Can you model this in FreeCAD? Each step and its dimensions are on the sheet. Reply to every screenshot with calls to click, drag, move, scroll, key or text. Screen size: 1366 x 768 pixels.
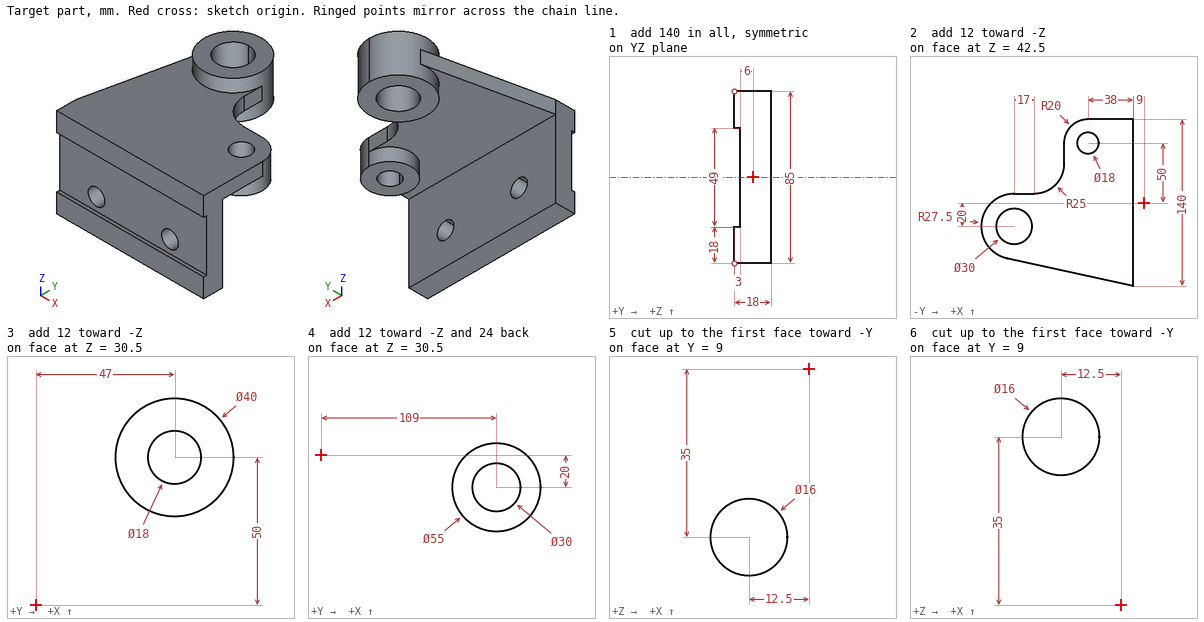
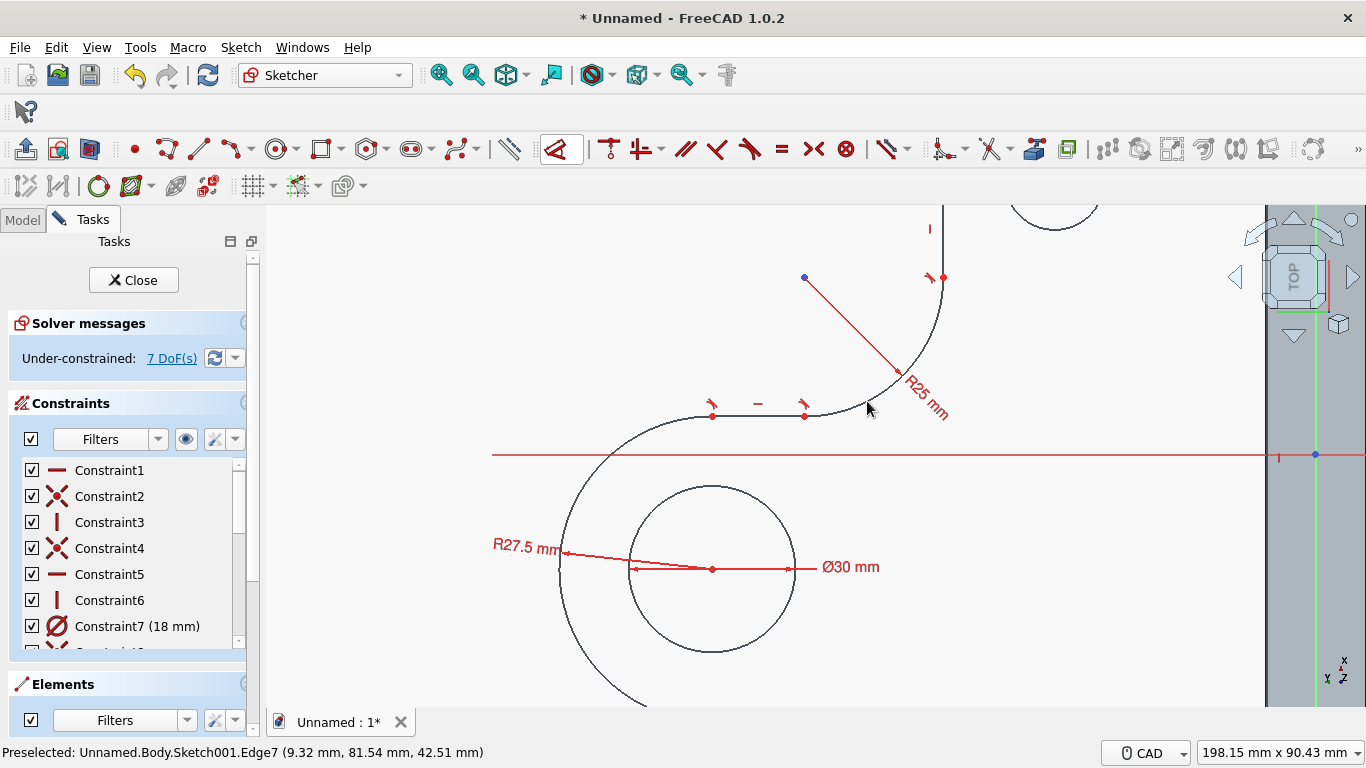
scroll(637, 457, down, 5)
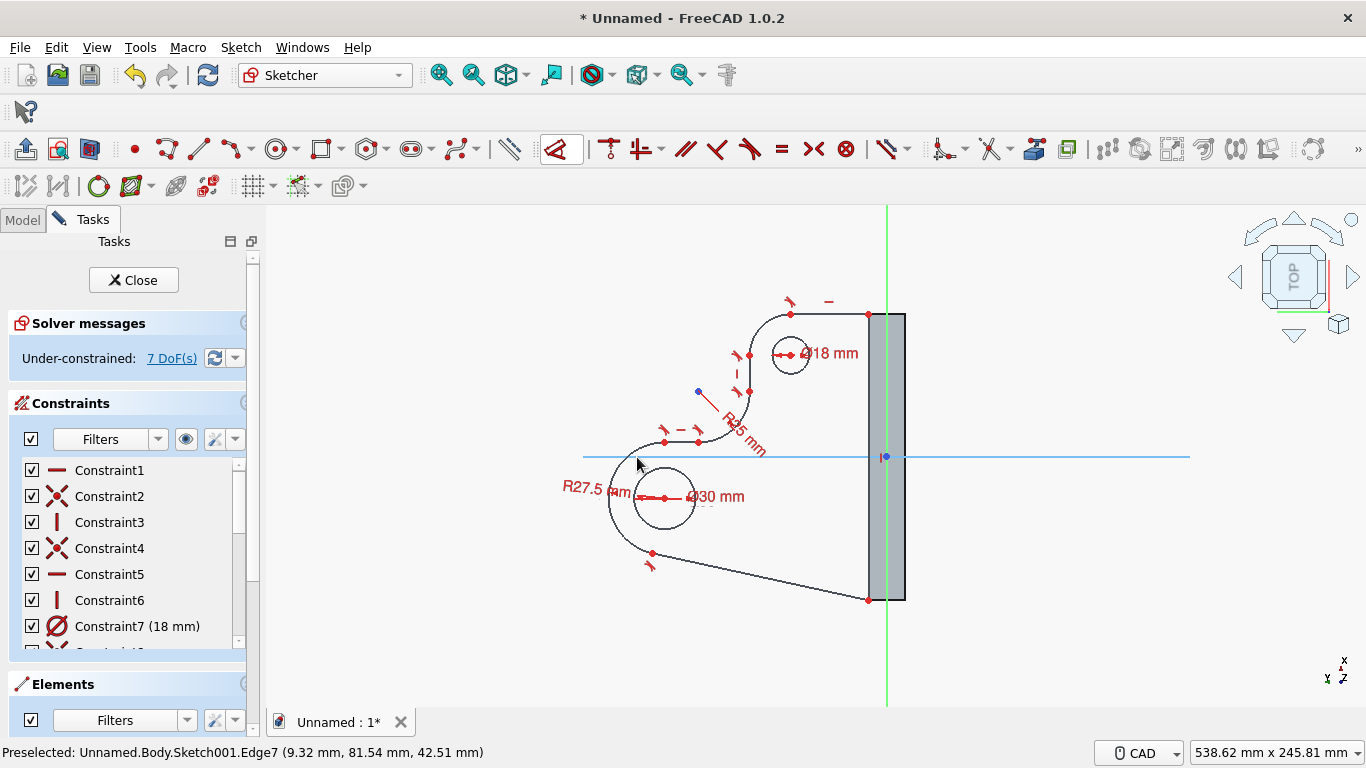
click(772, 319)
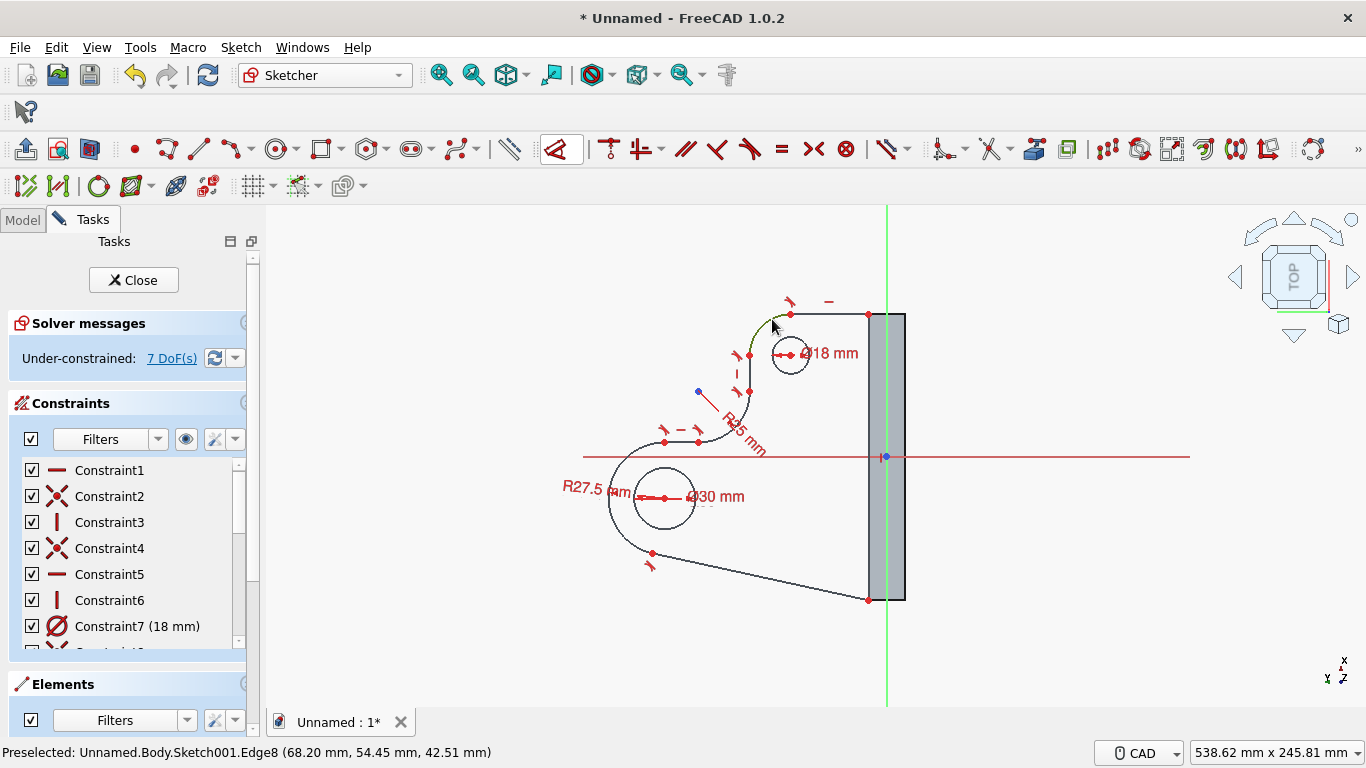
key(k)
key(r)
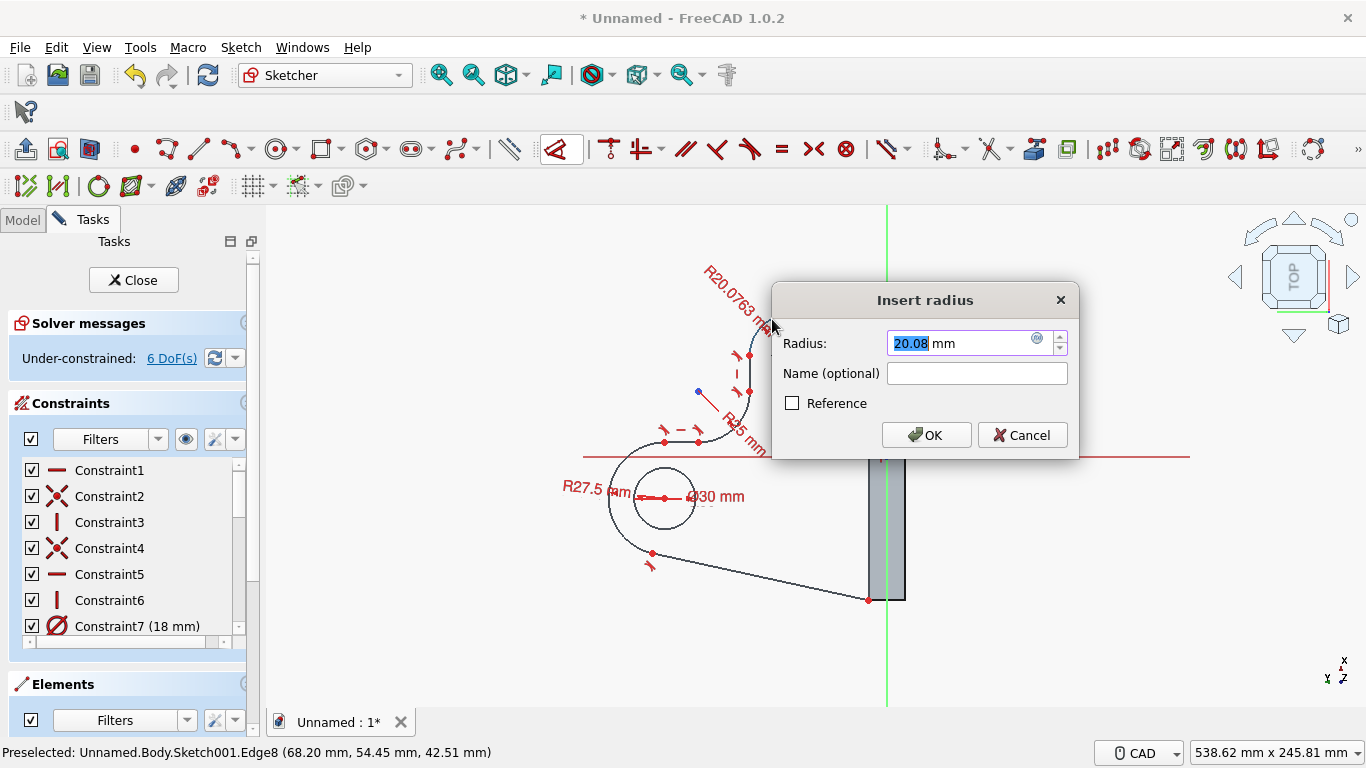
text(20)
key(Return)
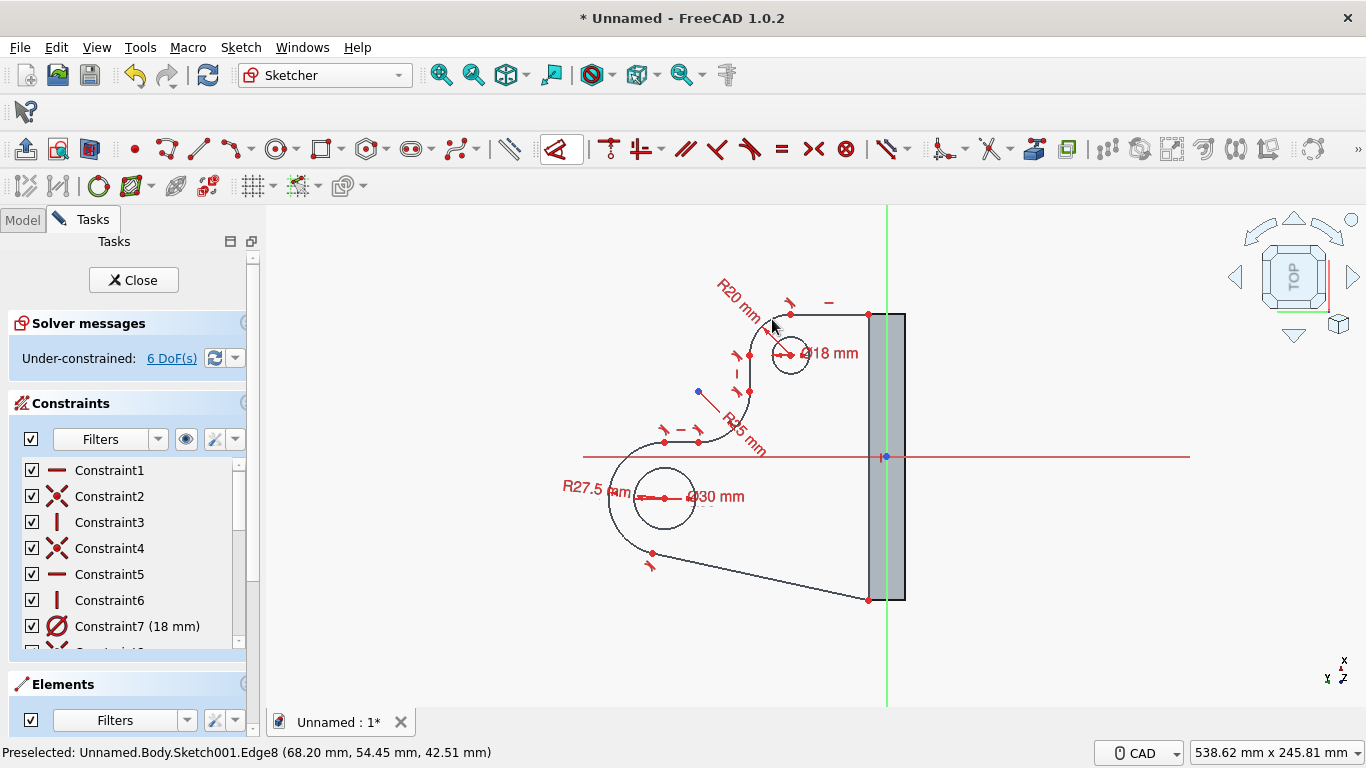
click(814, 315)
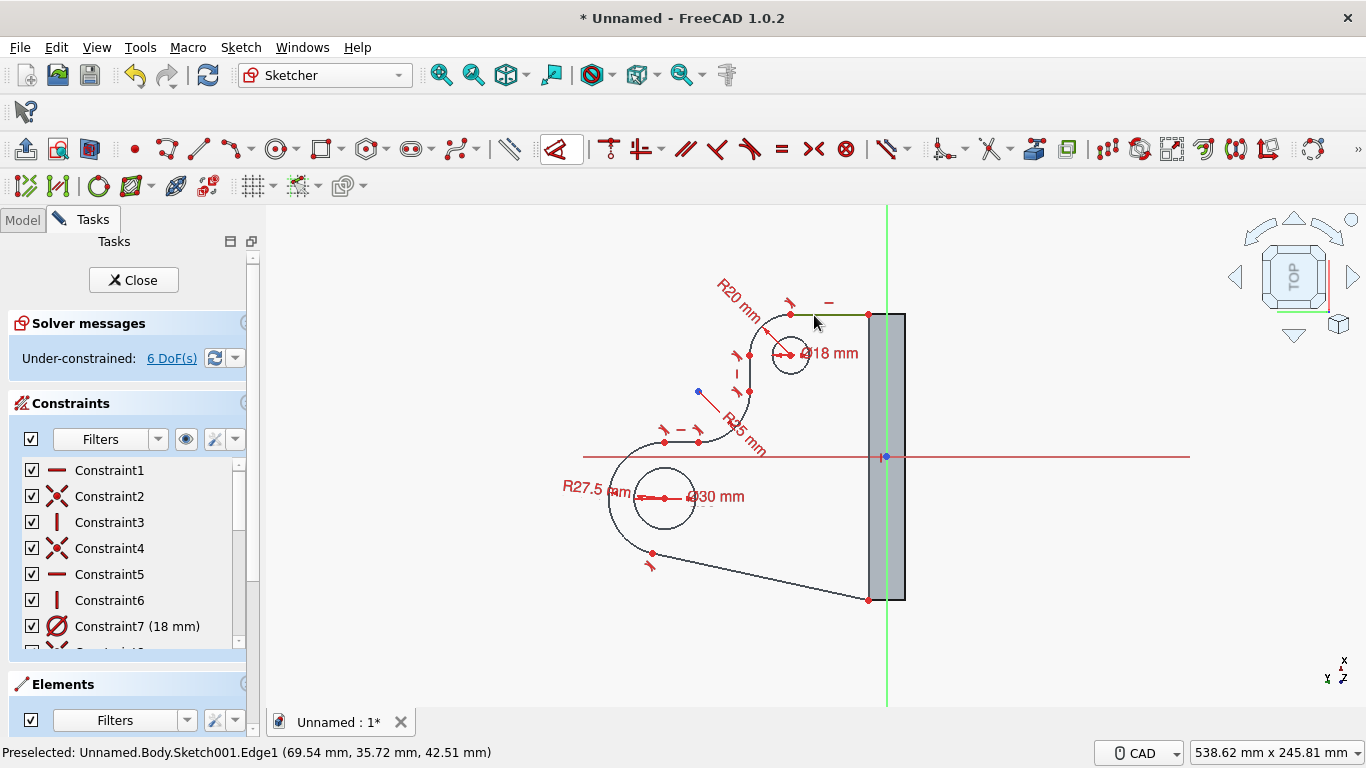
click(578, 150)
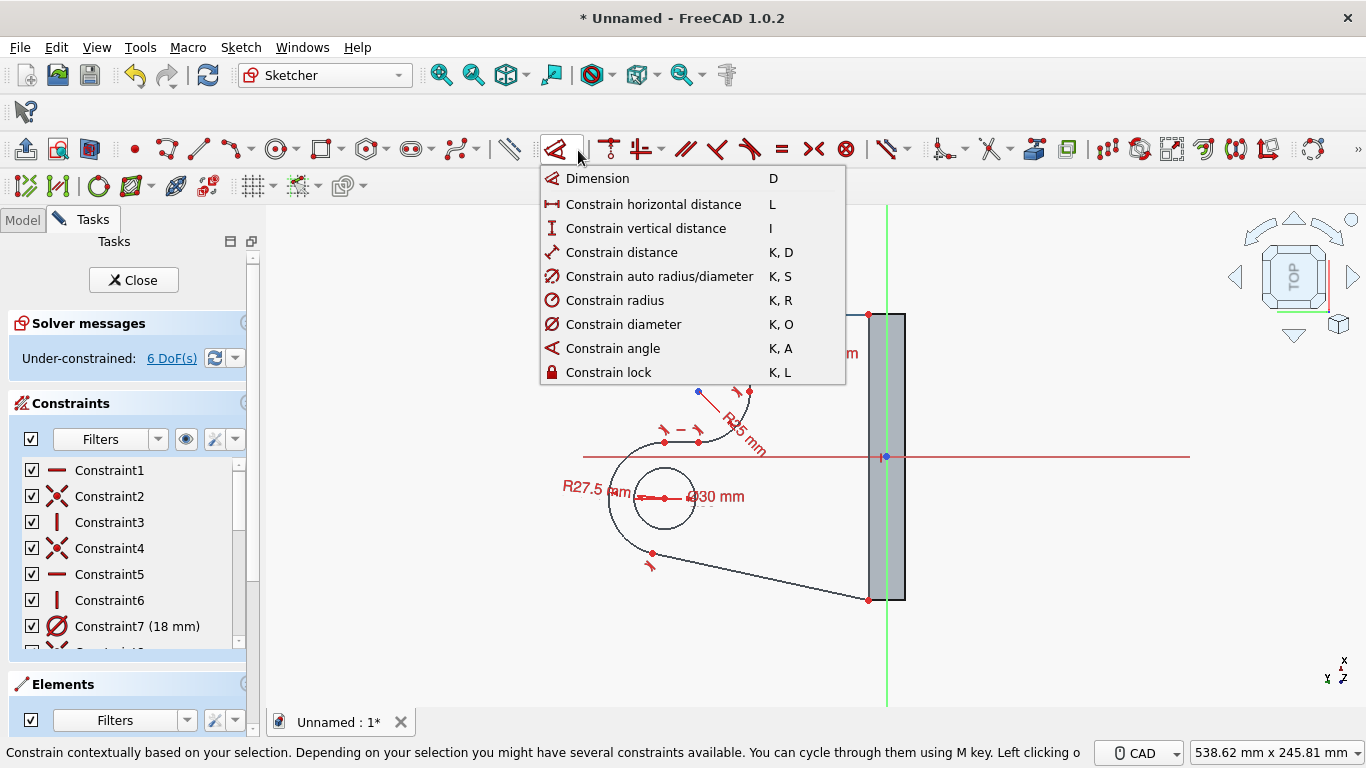
click(693, 204)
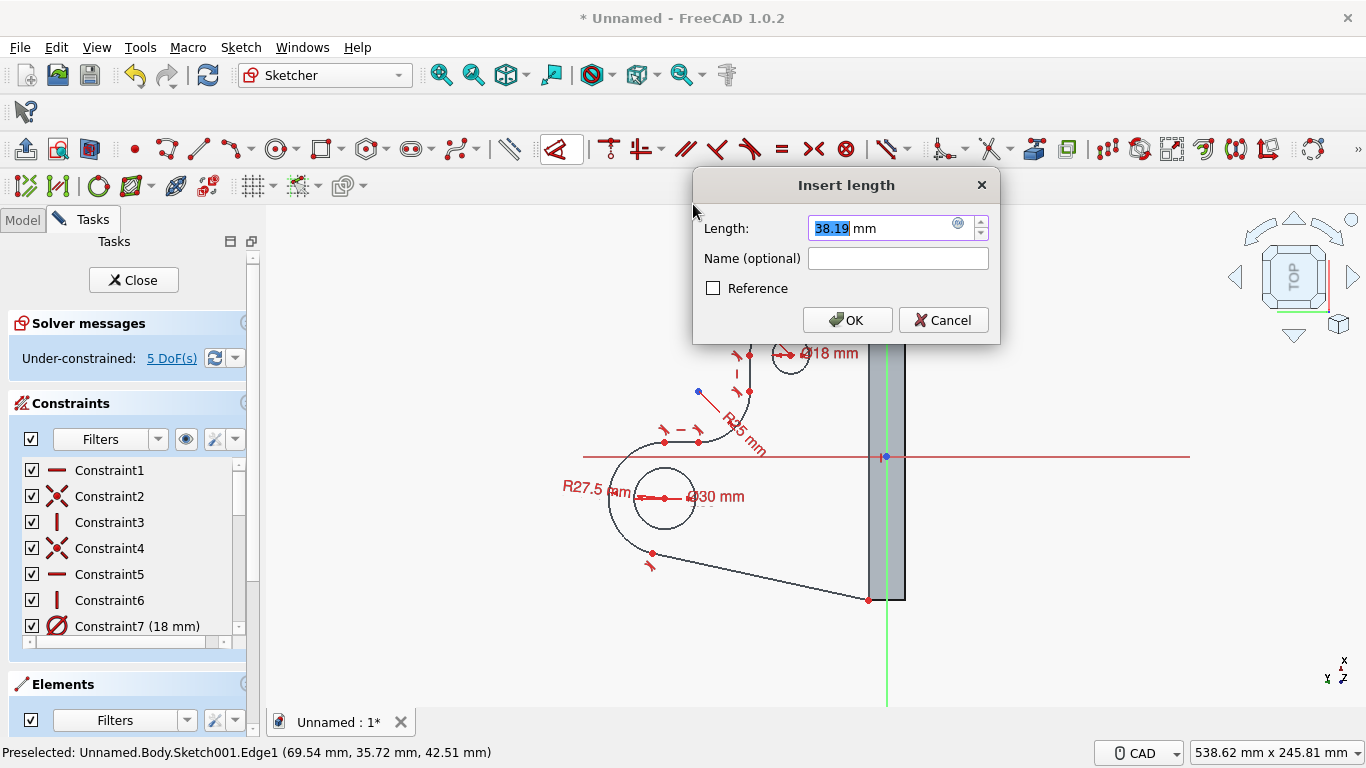
text(38)
key(Return)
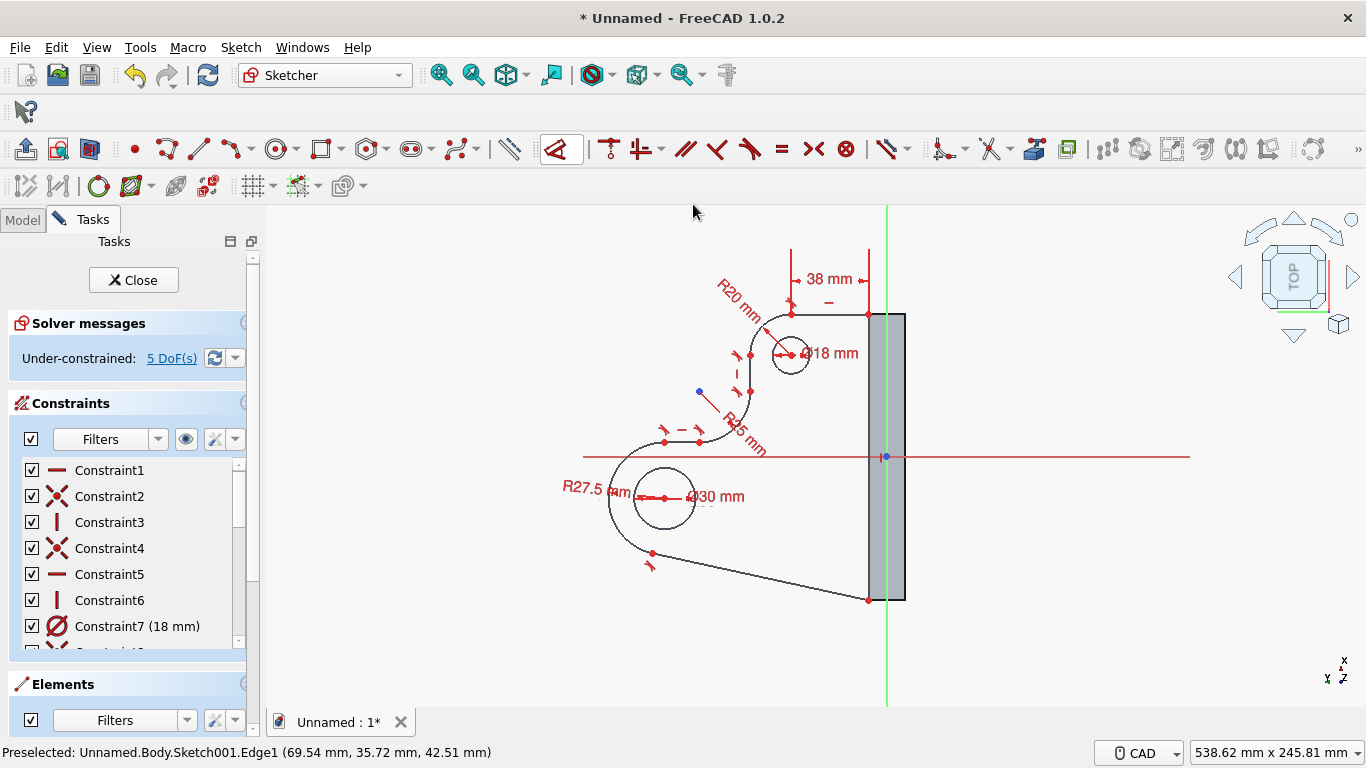
scroll(675, 442, up, 2)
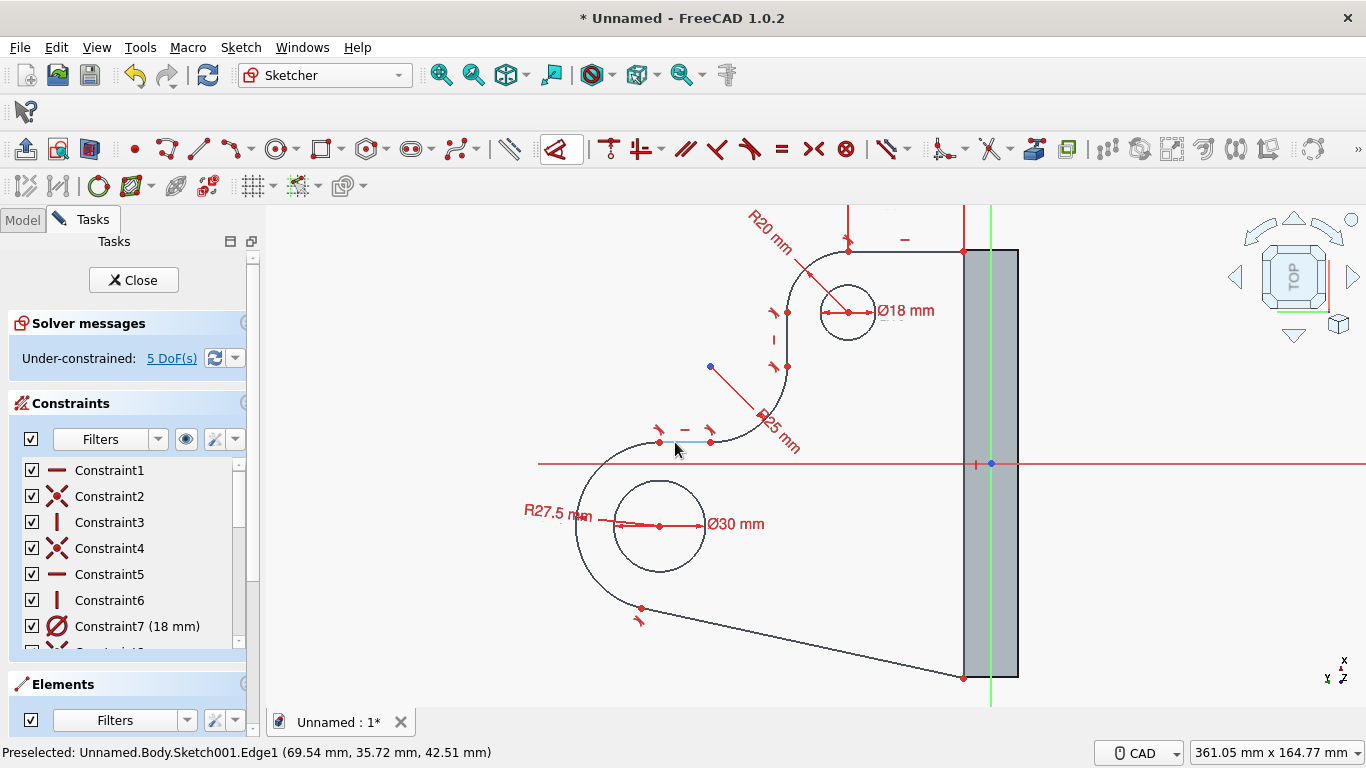
click(675, 442)